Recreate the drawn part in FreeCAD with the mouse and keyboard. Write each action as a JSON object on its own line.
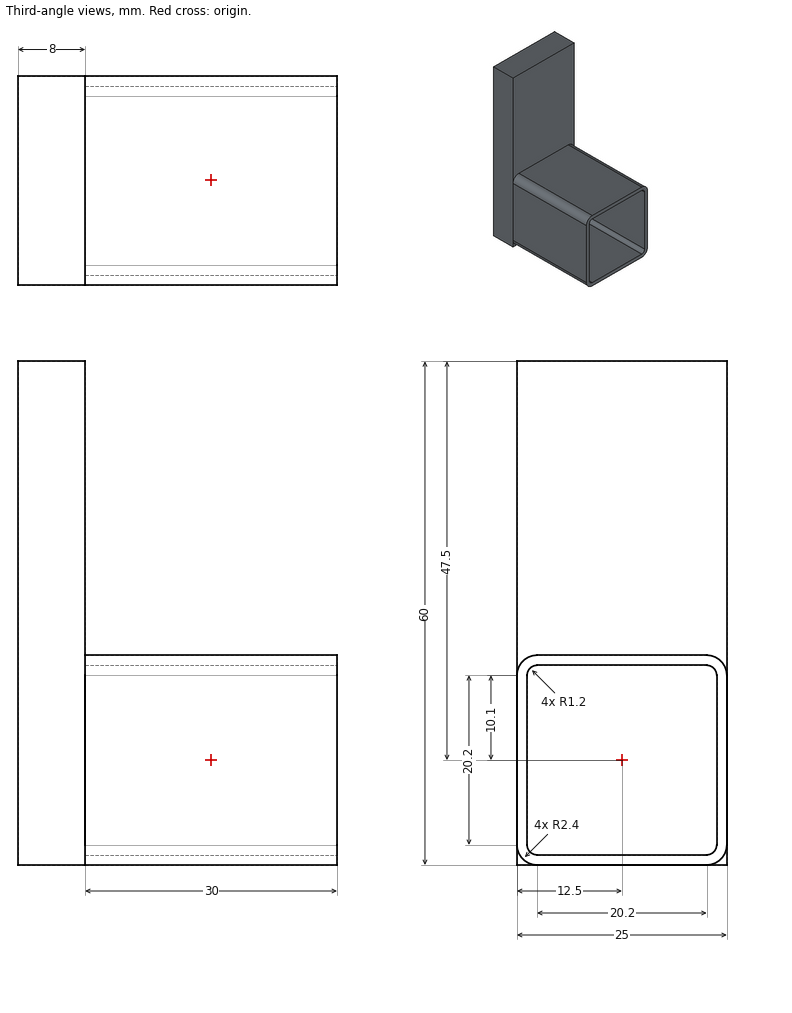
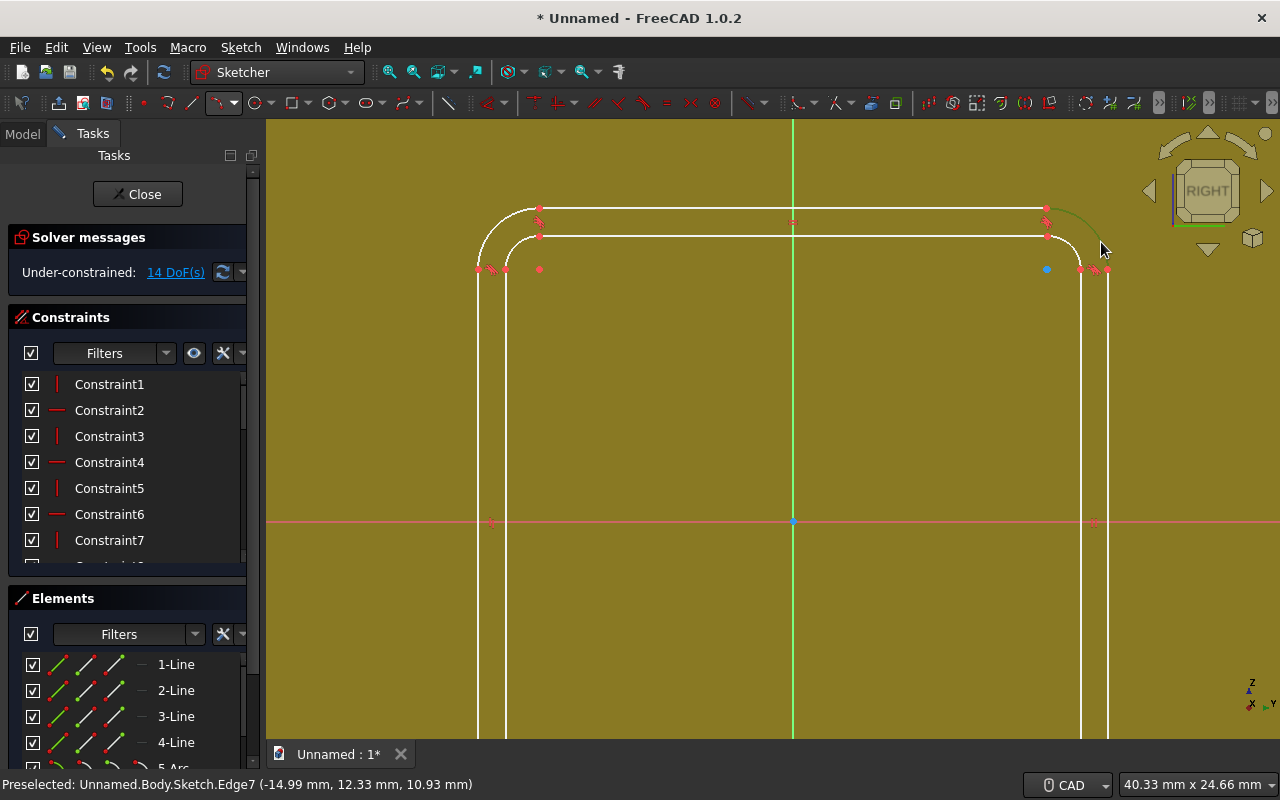
{"action": "left_click", "coordinate": [1077, 254]}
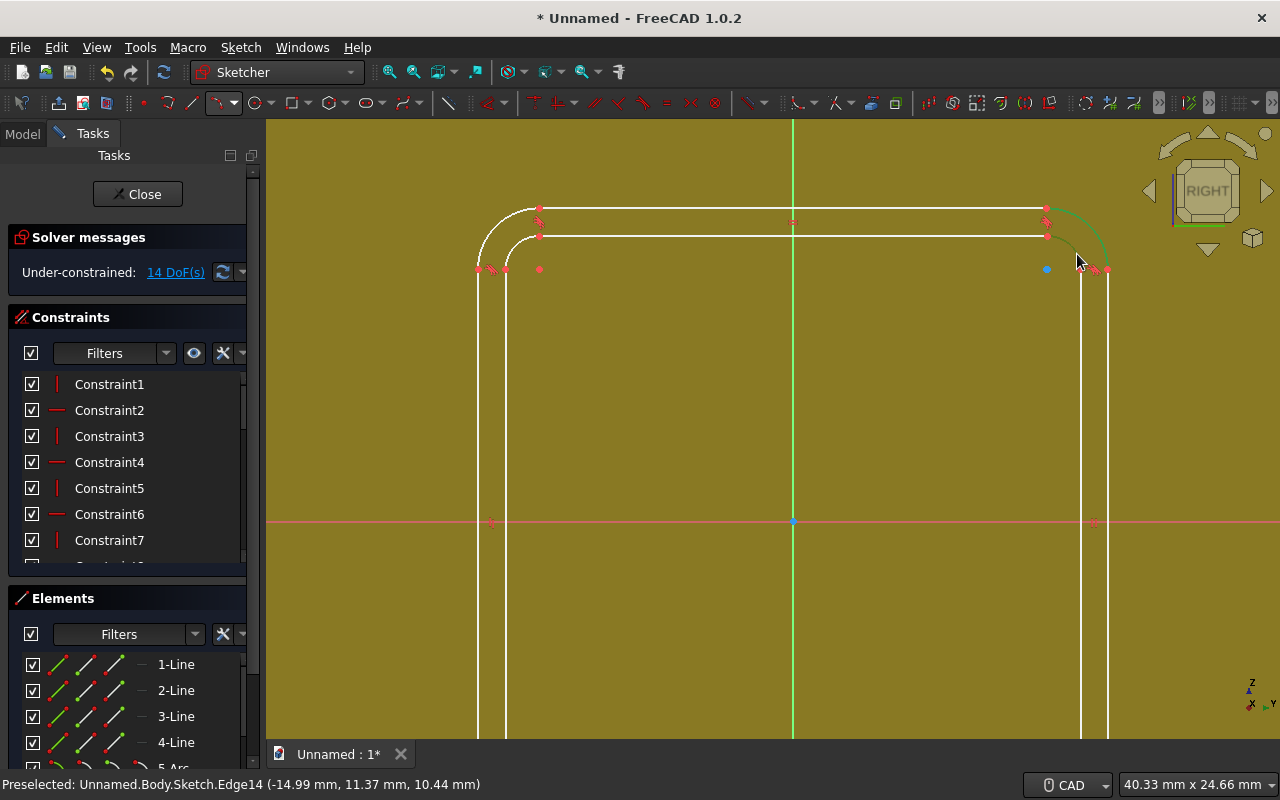
{"action": "key", "text": "c"}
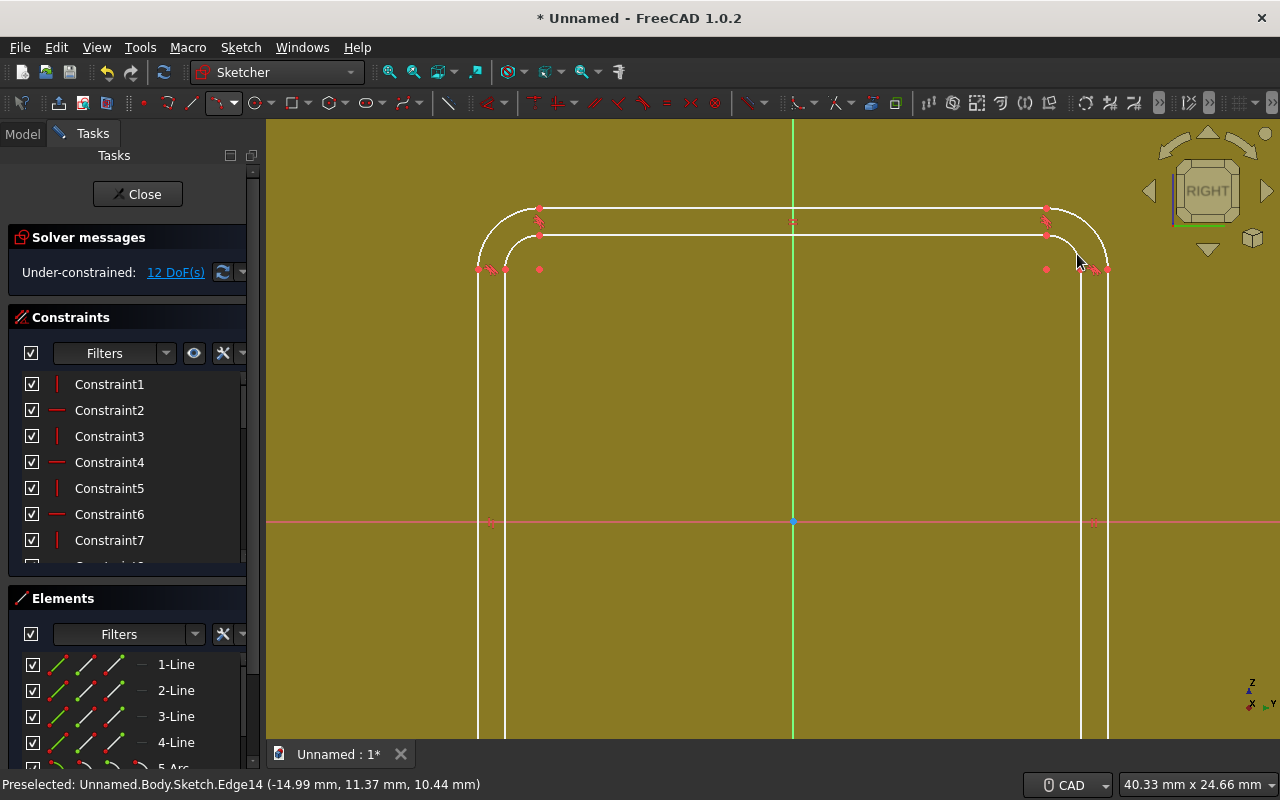
{"action": "scroll", "coordinate": [524, 241], "scroll_direction": "down", "scroll_amount": 2}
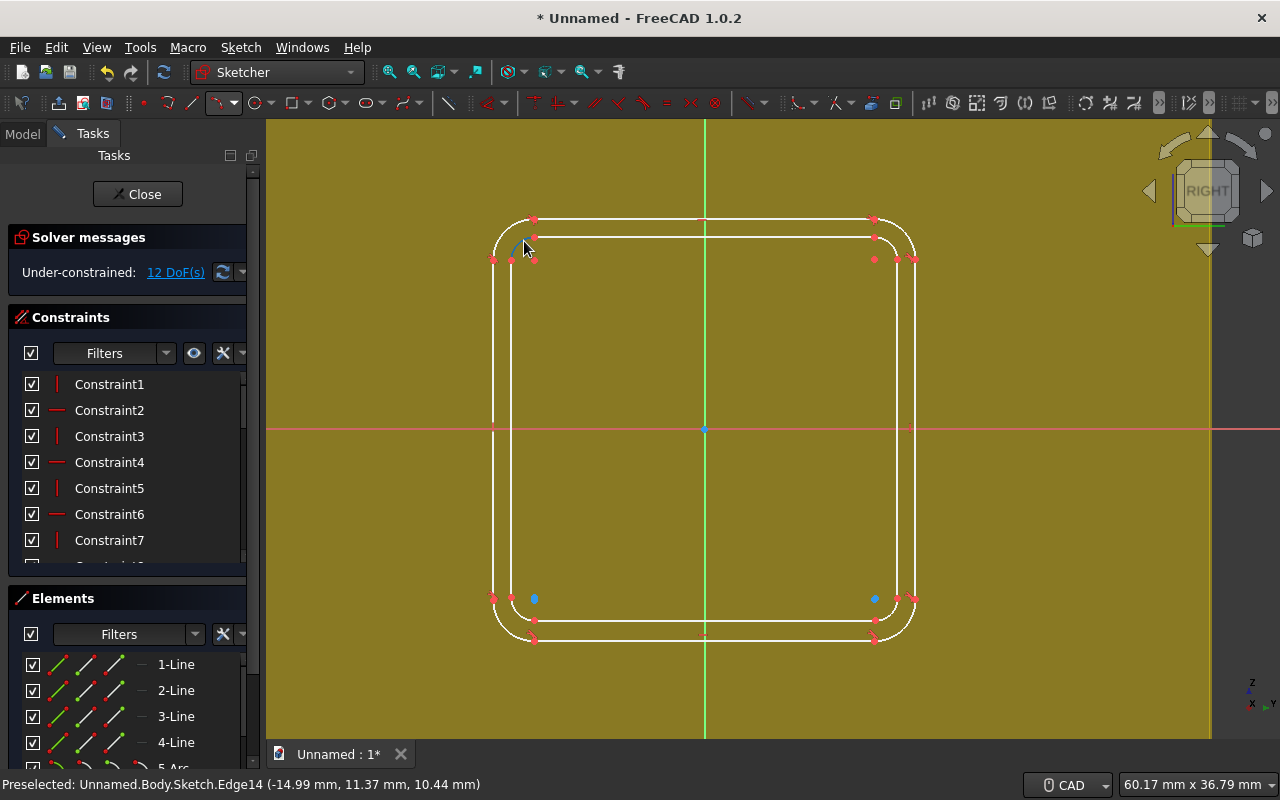
{"action": "left_click", "coordinate": [893, 637]}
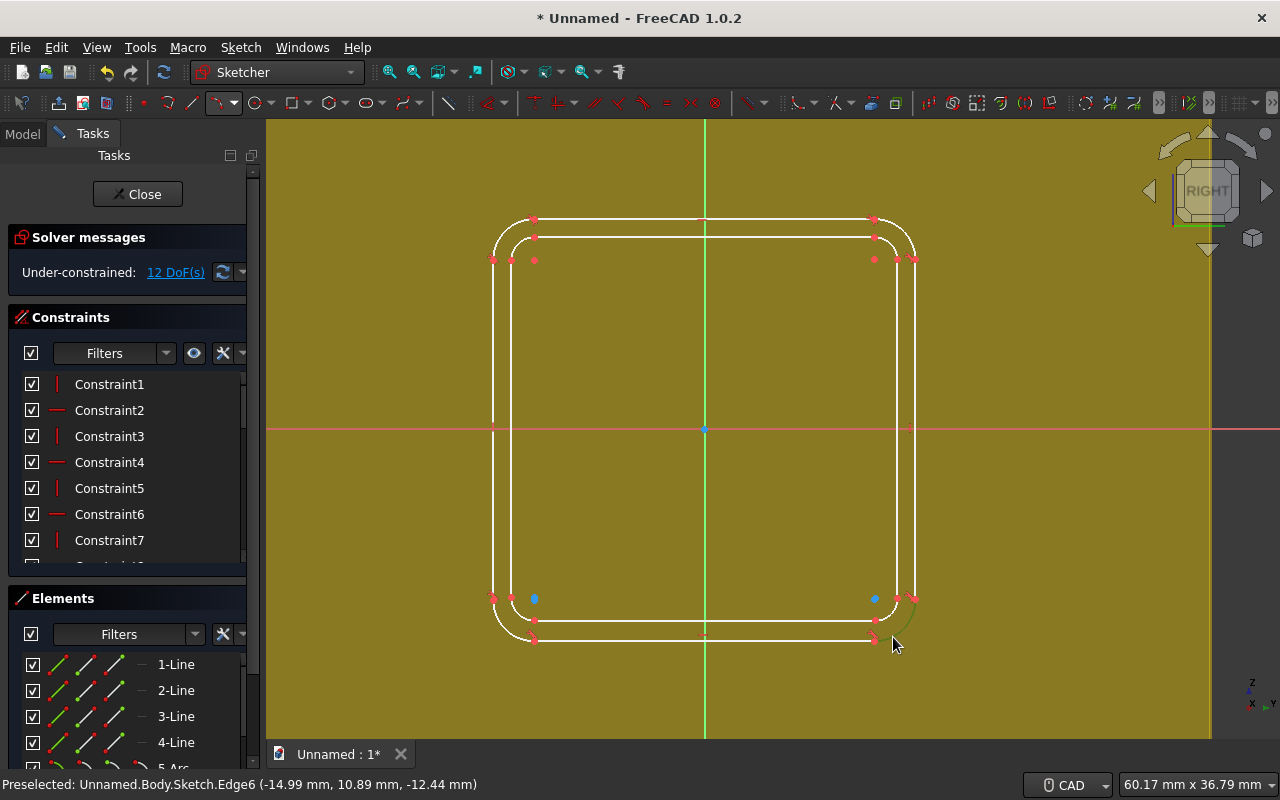
{"action": "scroll", "coordinate": [885, 618], "scroll_direction": "up", "scroll_amount": 2}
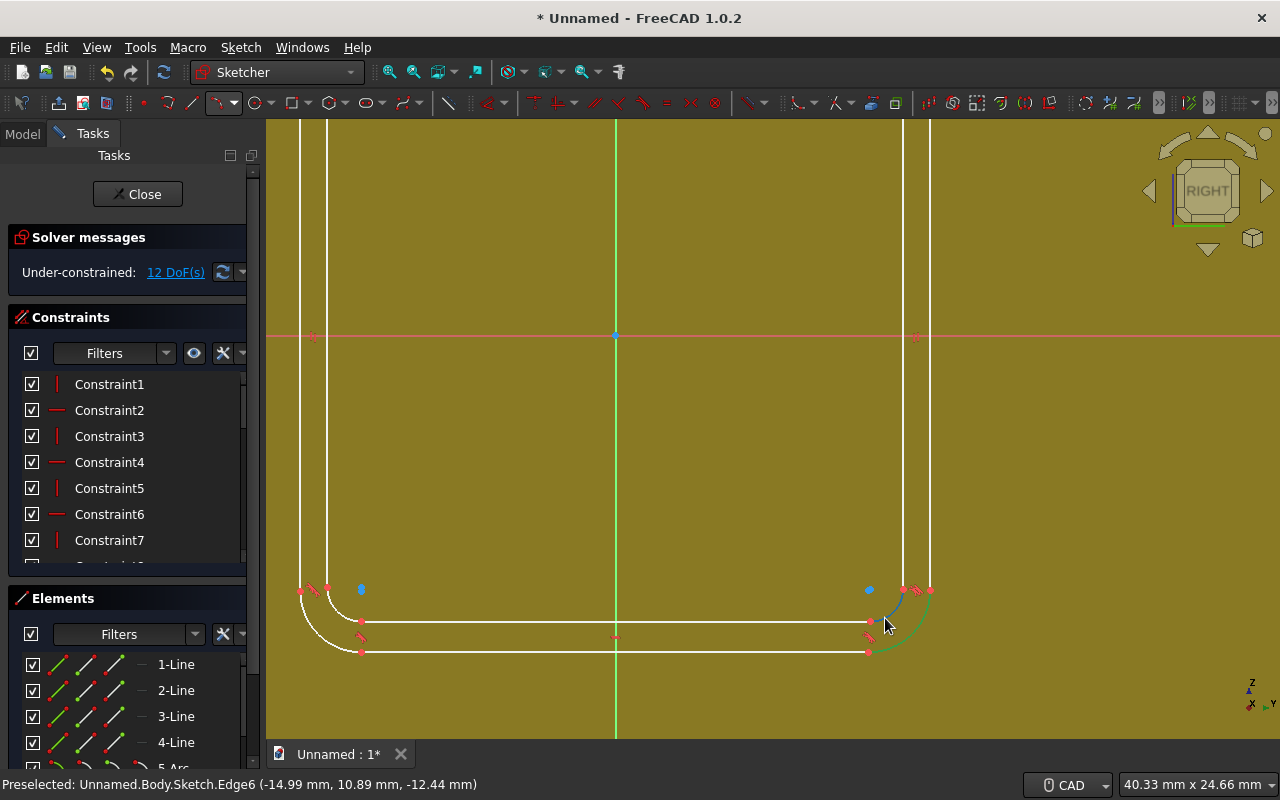
{"action": "left_click", "coordinate": [885, 618]}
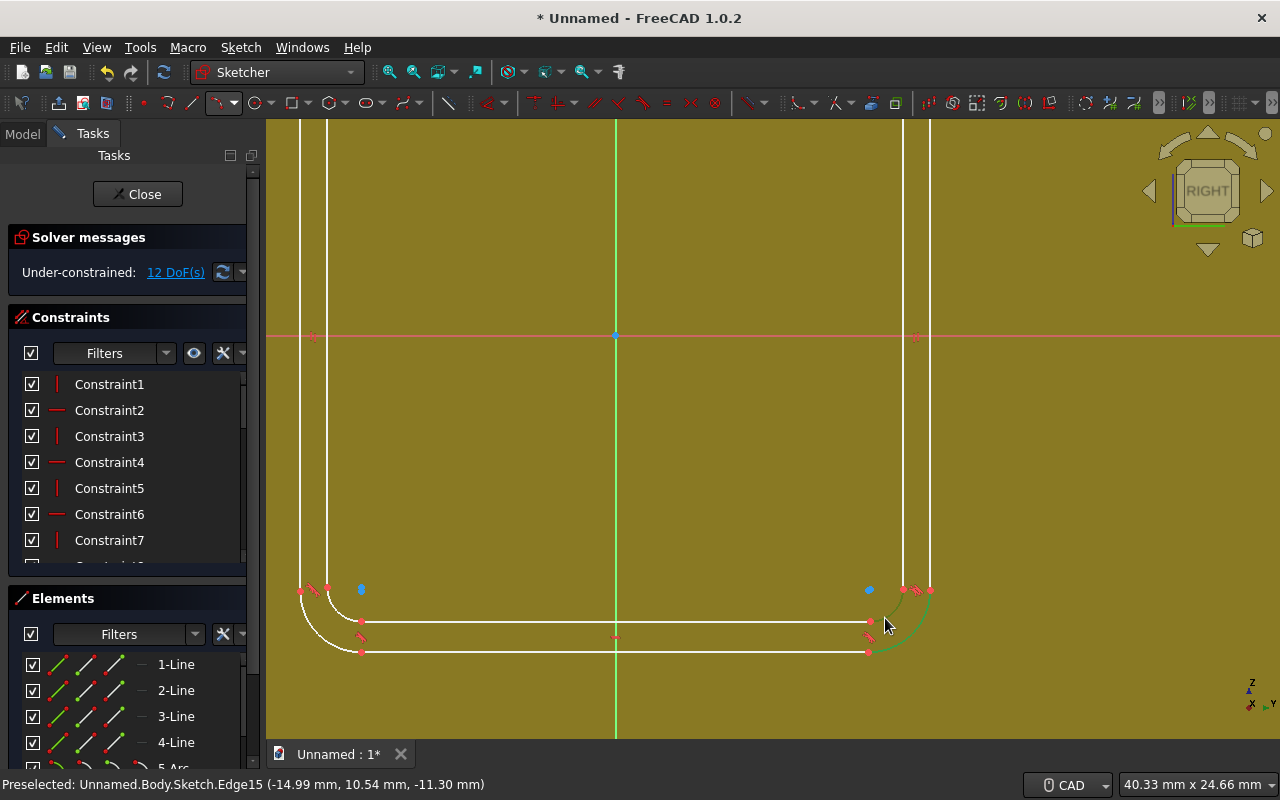
{"action": "left_click", "coordinate": [534, 104]}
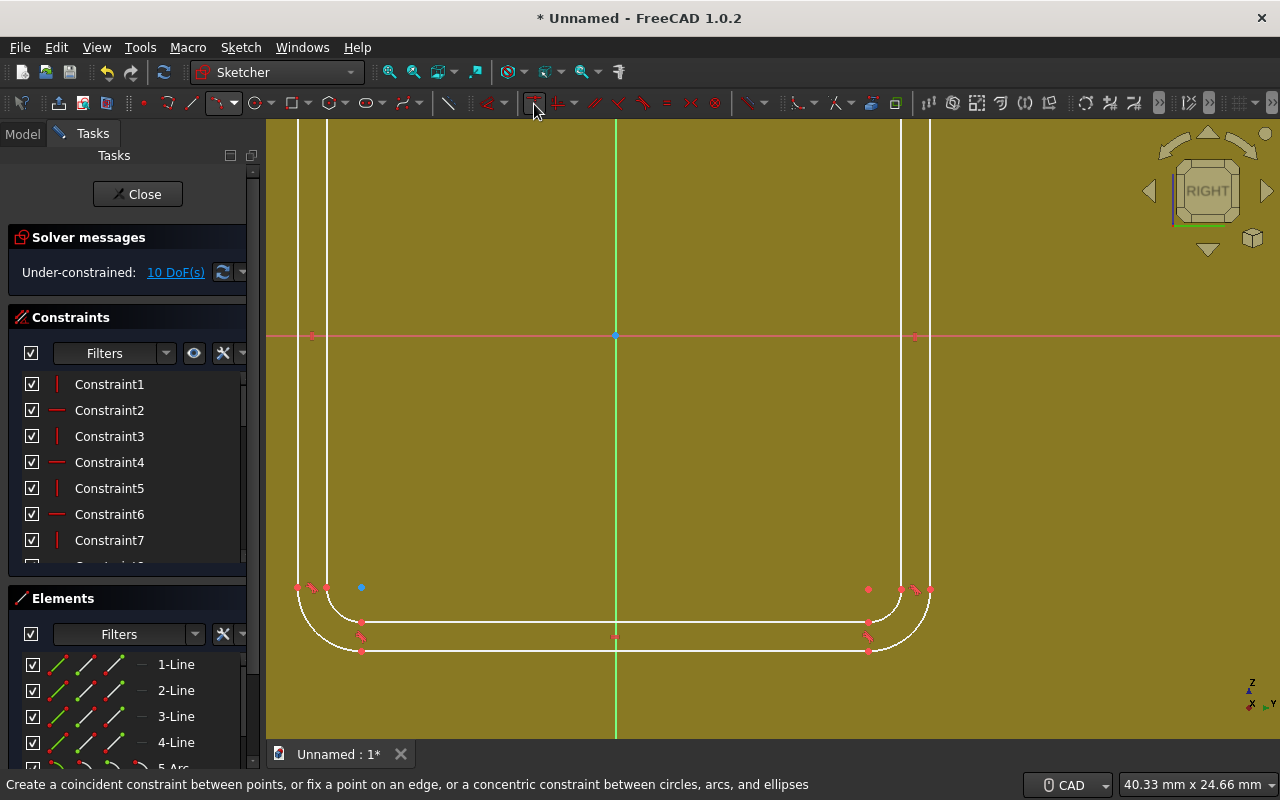
{"action": "left_click", "coordinate": [305, 616]}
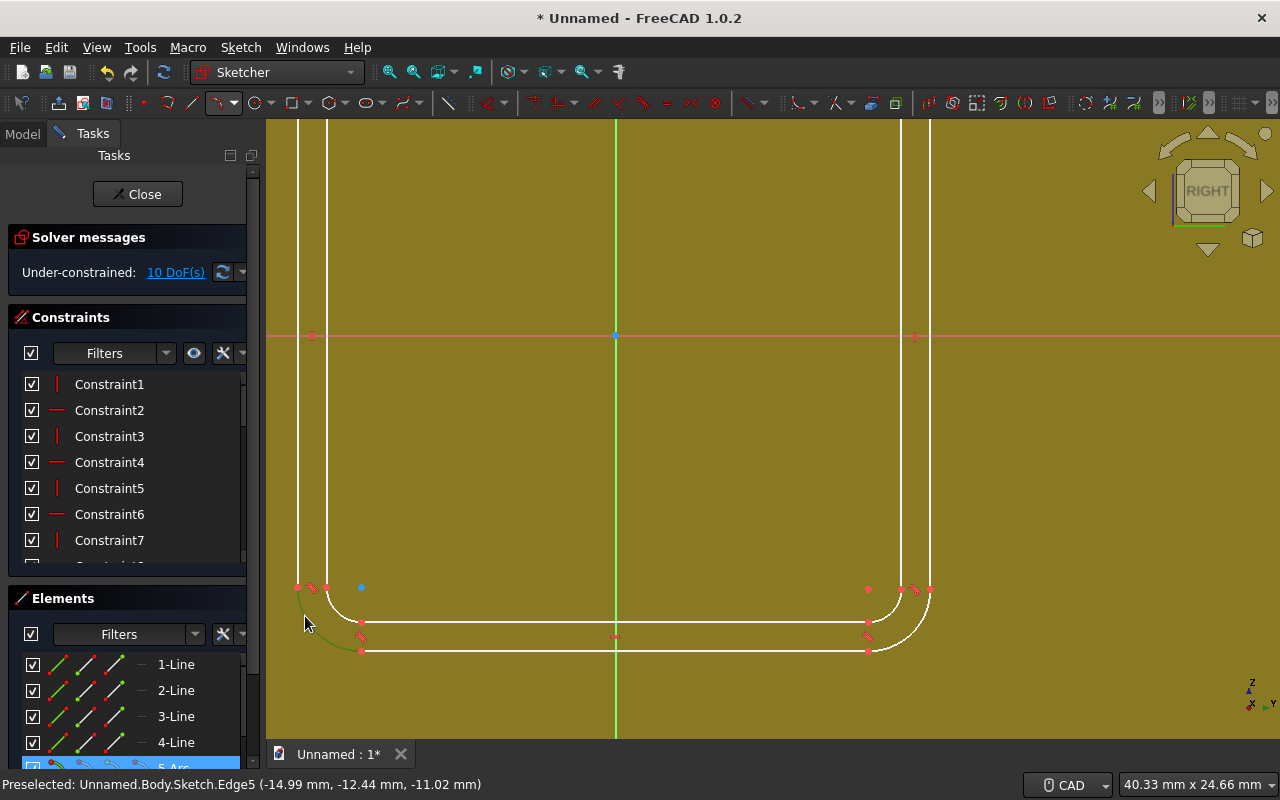
{"action": "left_click", "coordinate": [897, 644]}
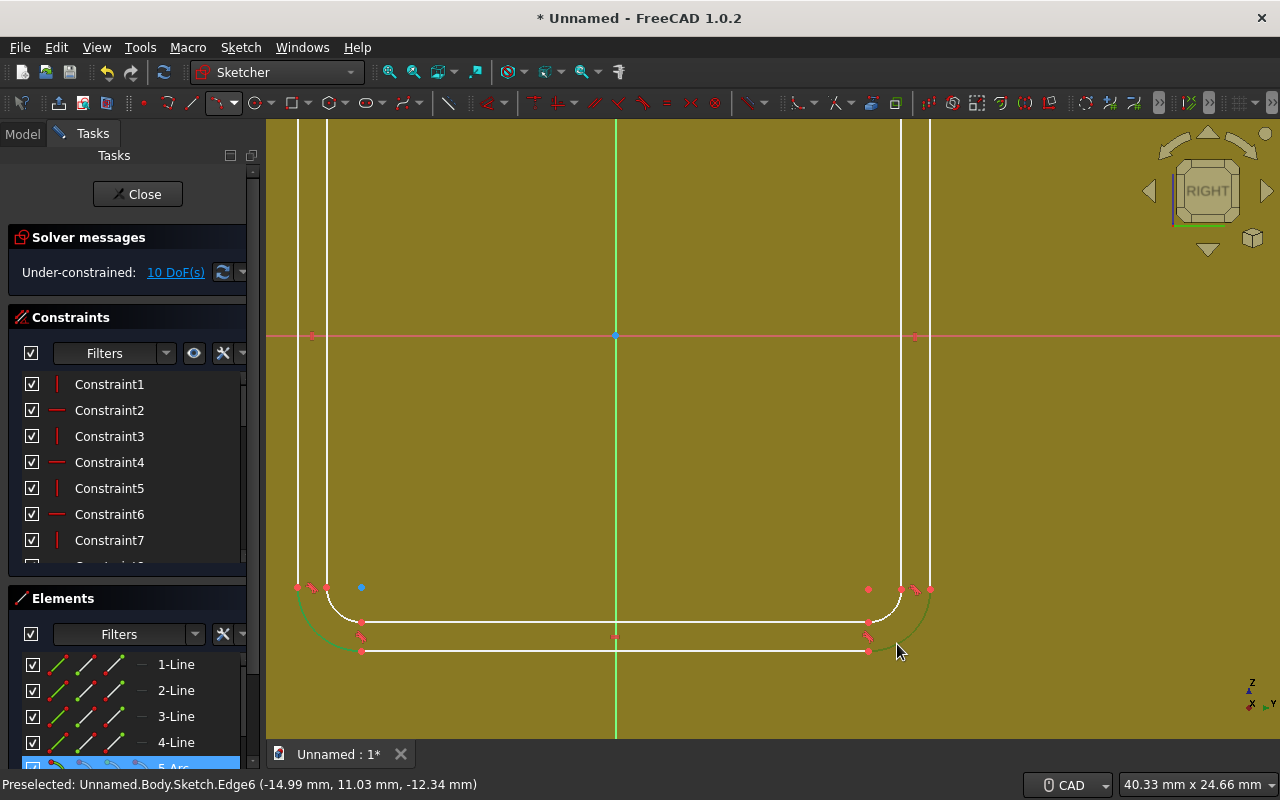
{"action": "scroll", "coordinate": [885, 618], "scroll_direction": "down", "scroll_amount": 2}